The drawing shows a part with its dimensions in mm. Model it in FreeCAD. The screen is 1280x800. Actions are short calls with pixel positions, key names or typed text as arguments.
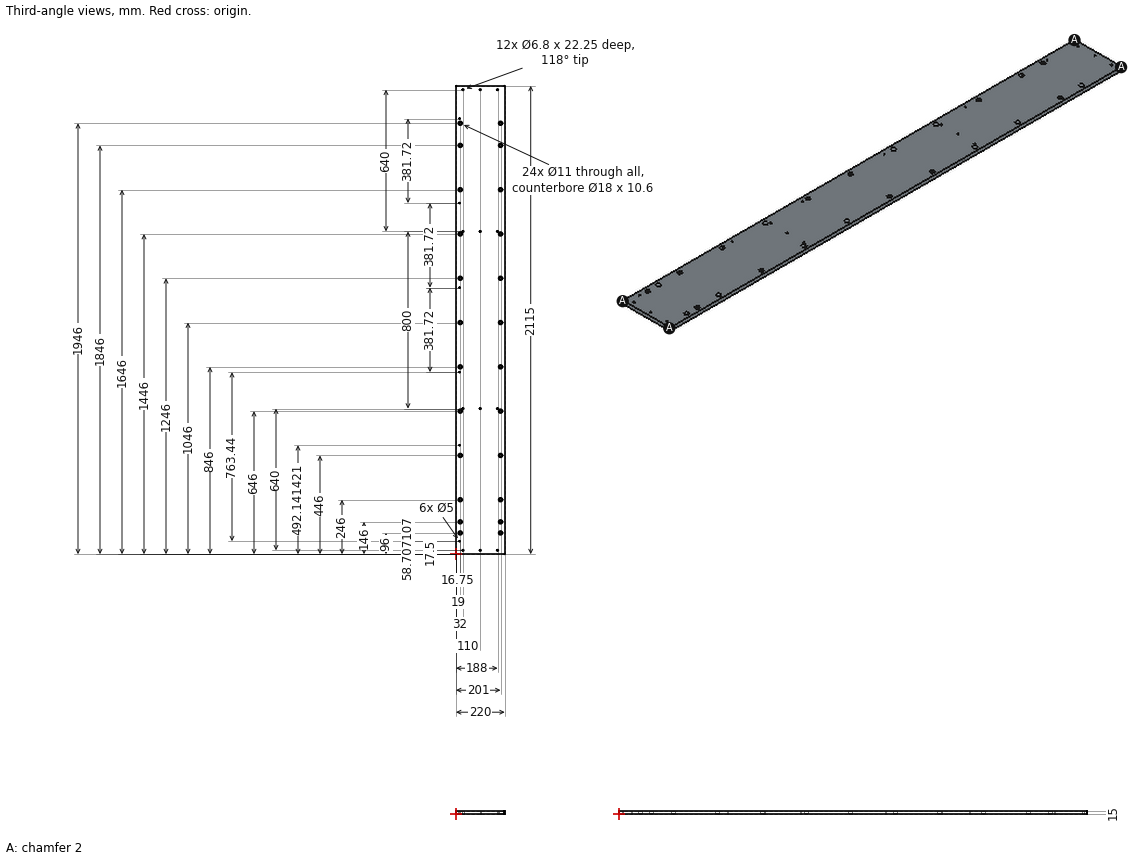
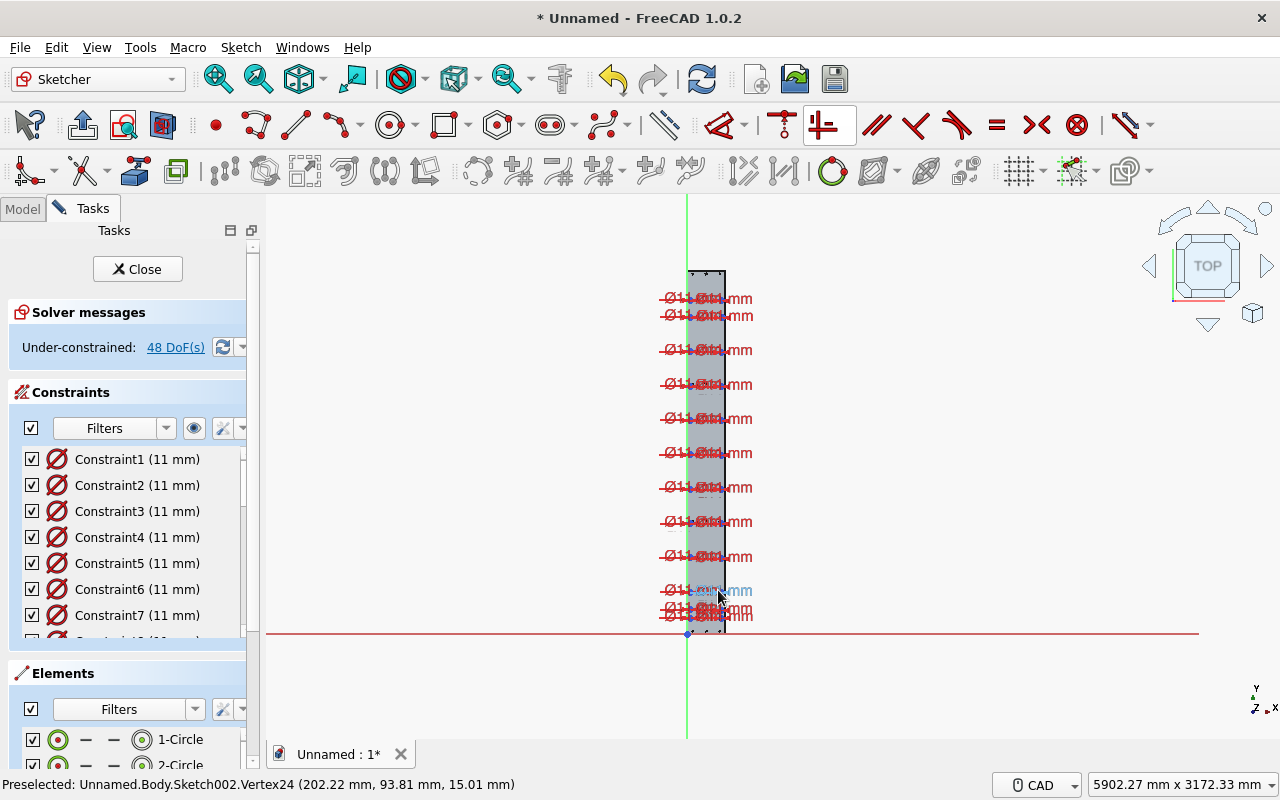
click(690, 300)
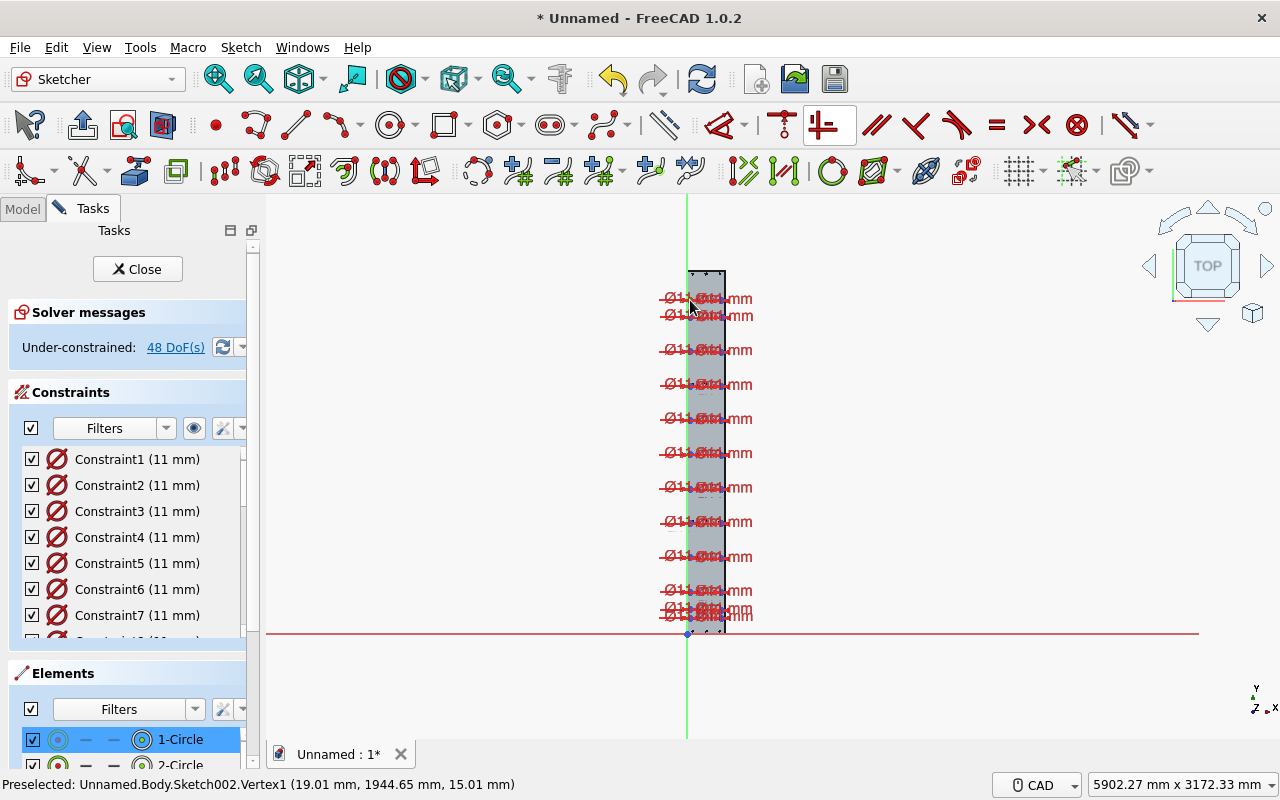
click(721, 301)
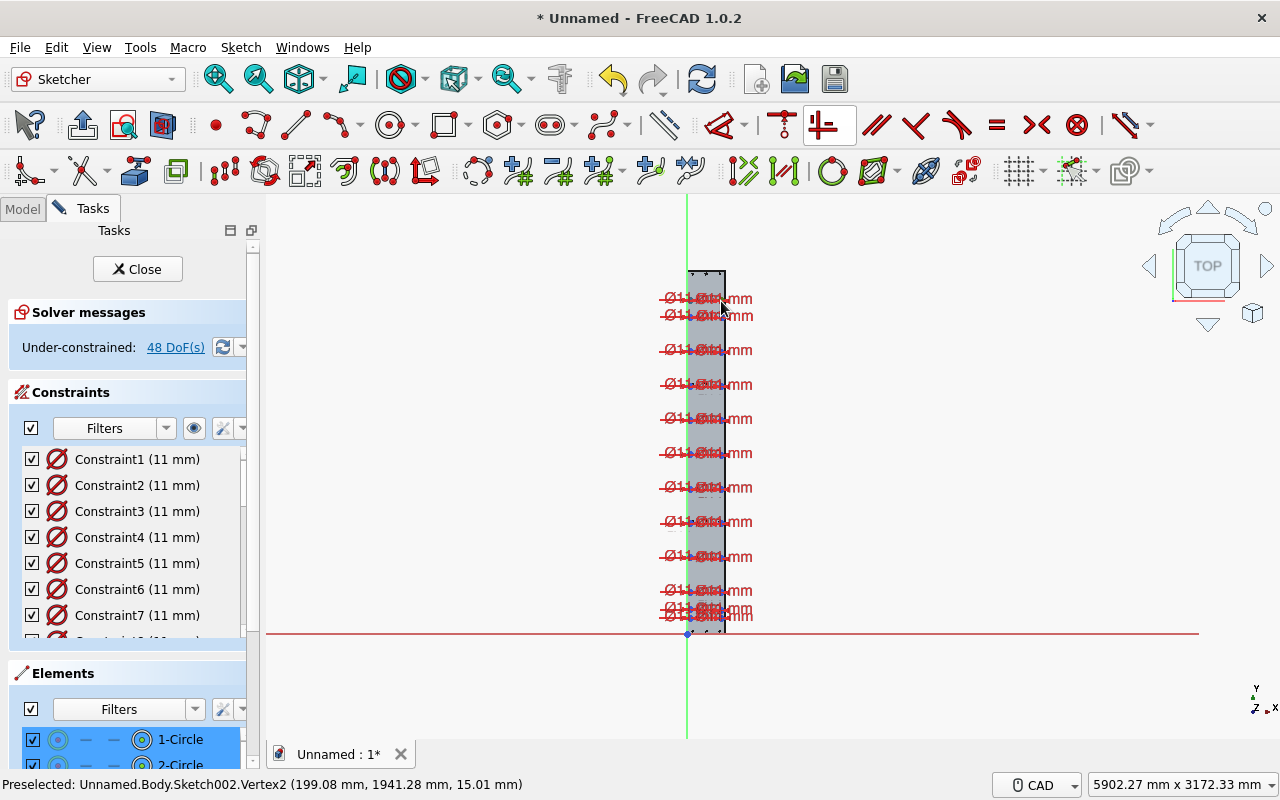
key(h)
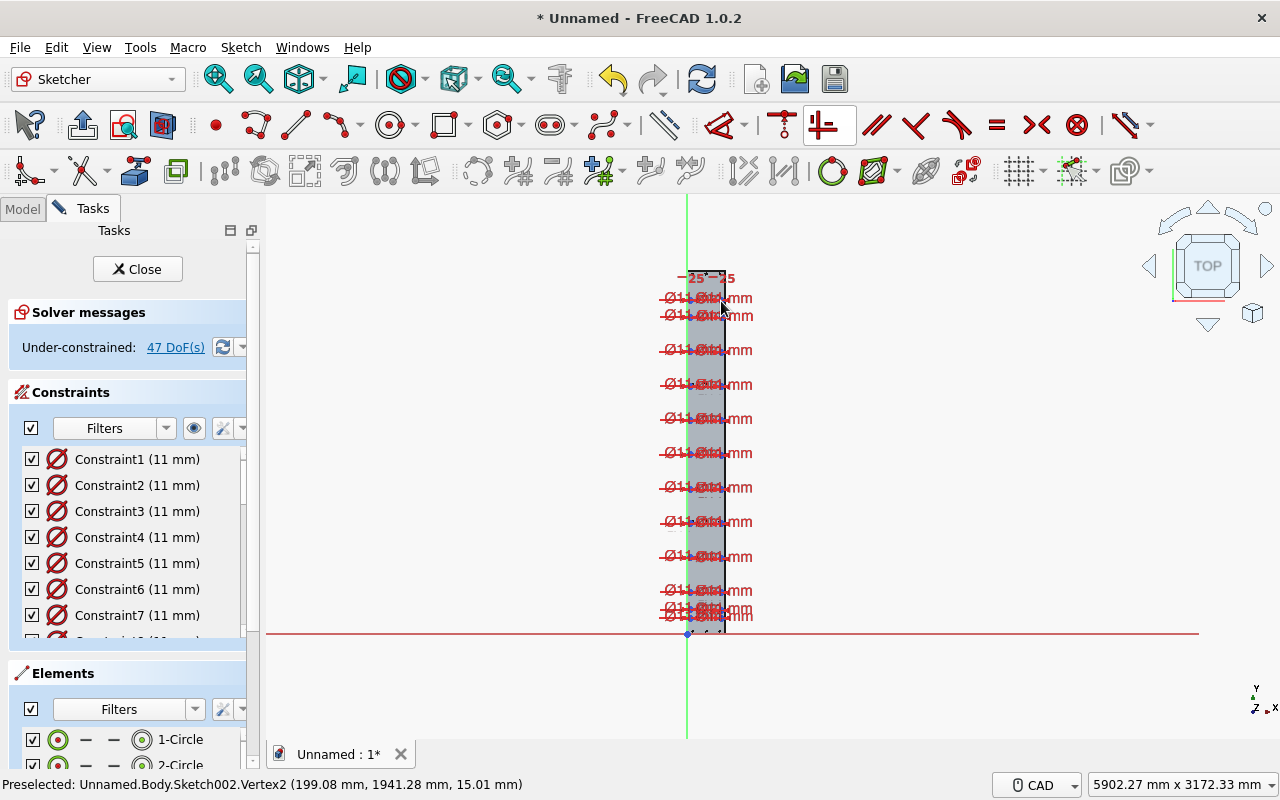
click(690, 300)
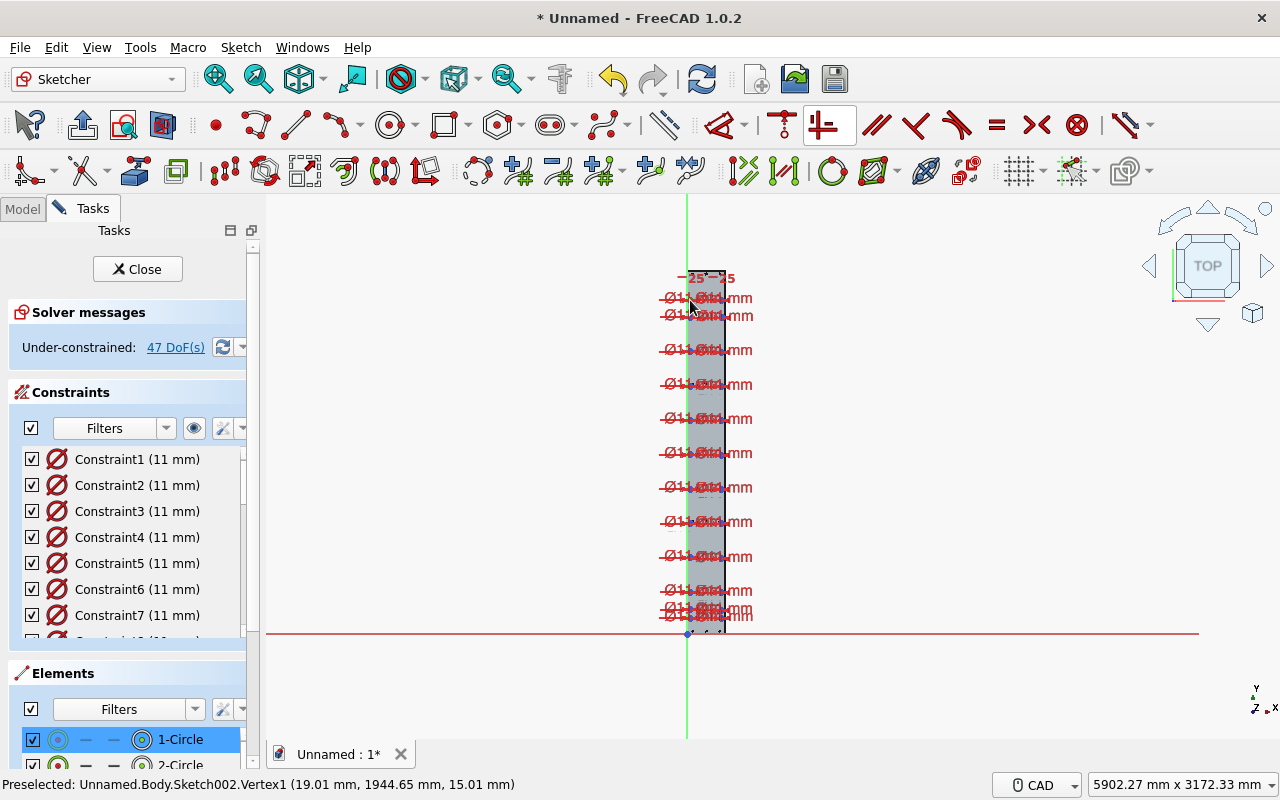
click(690, 317)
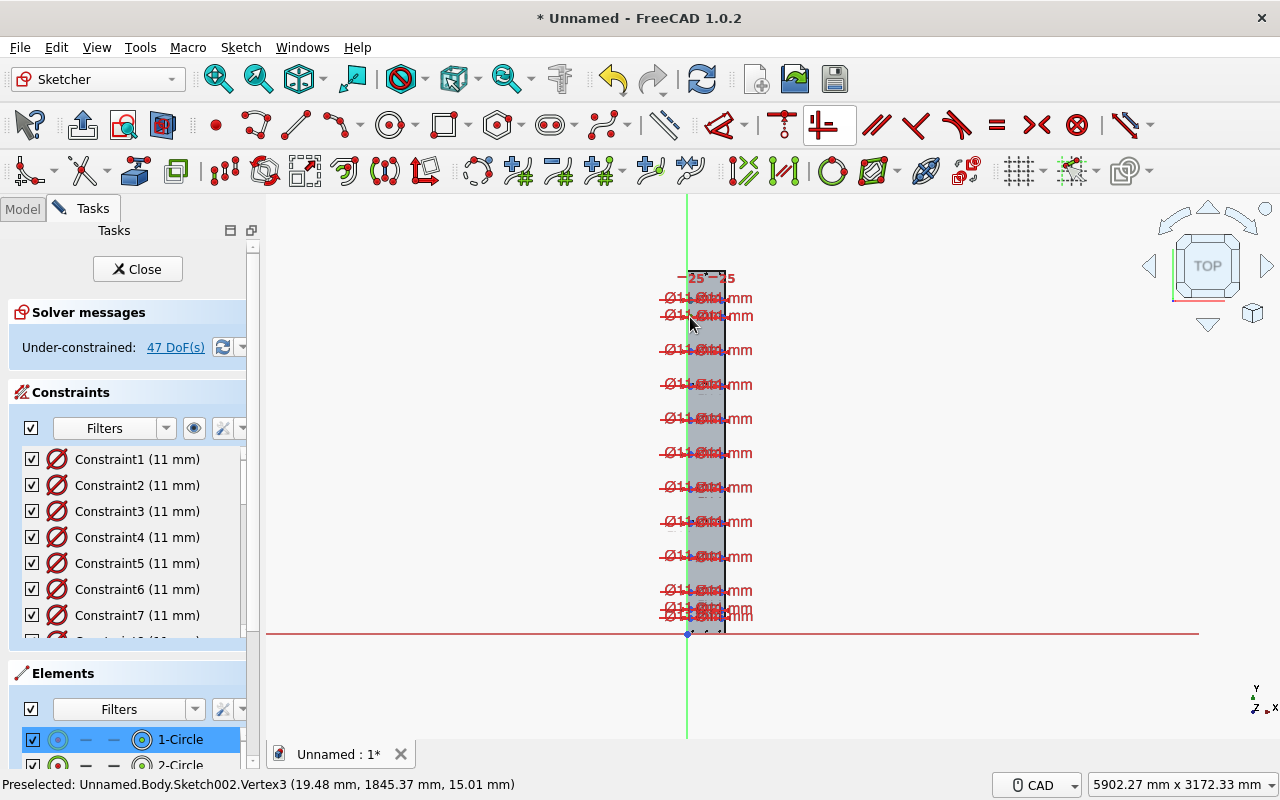
click(850, 126)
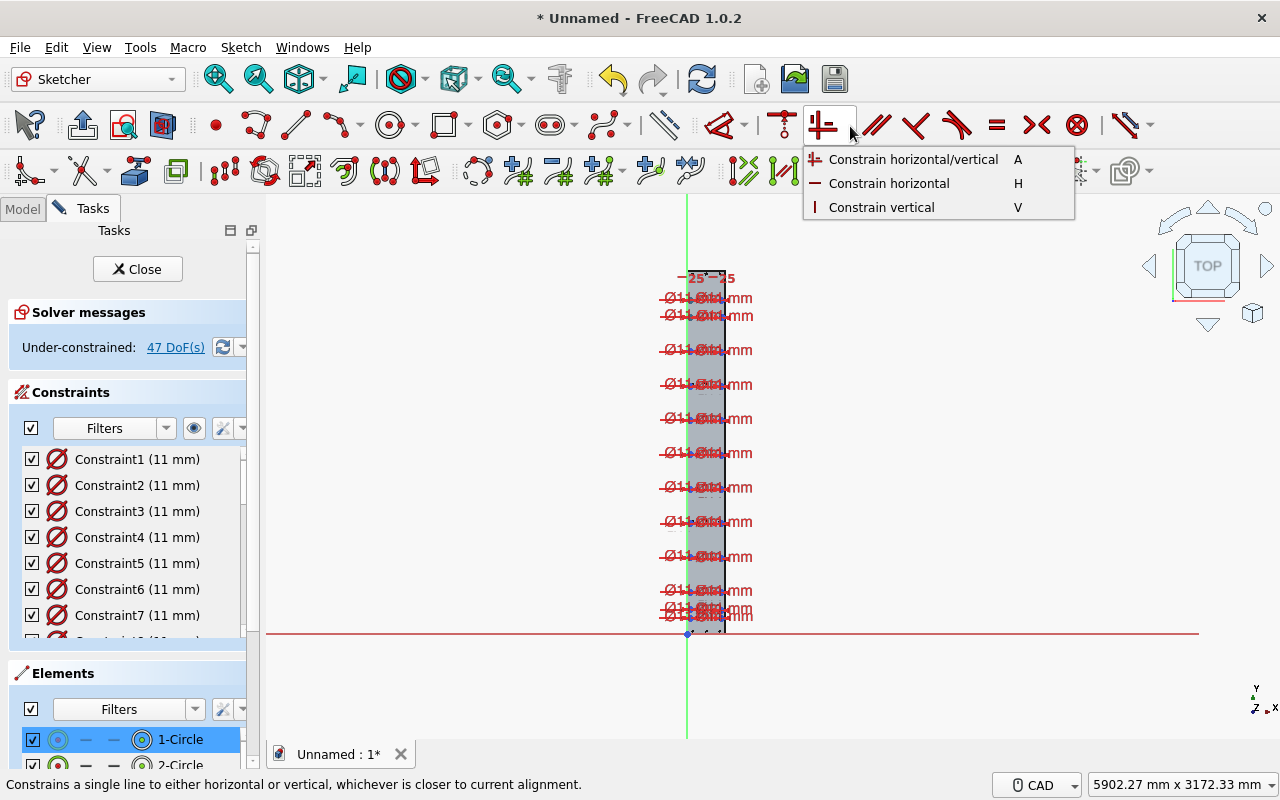
click(939, 207)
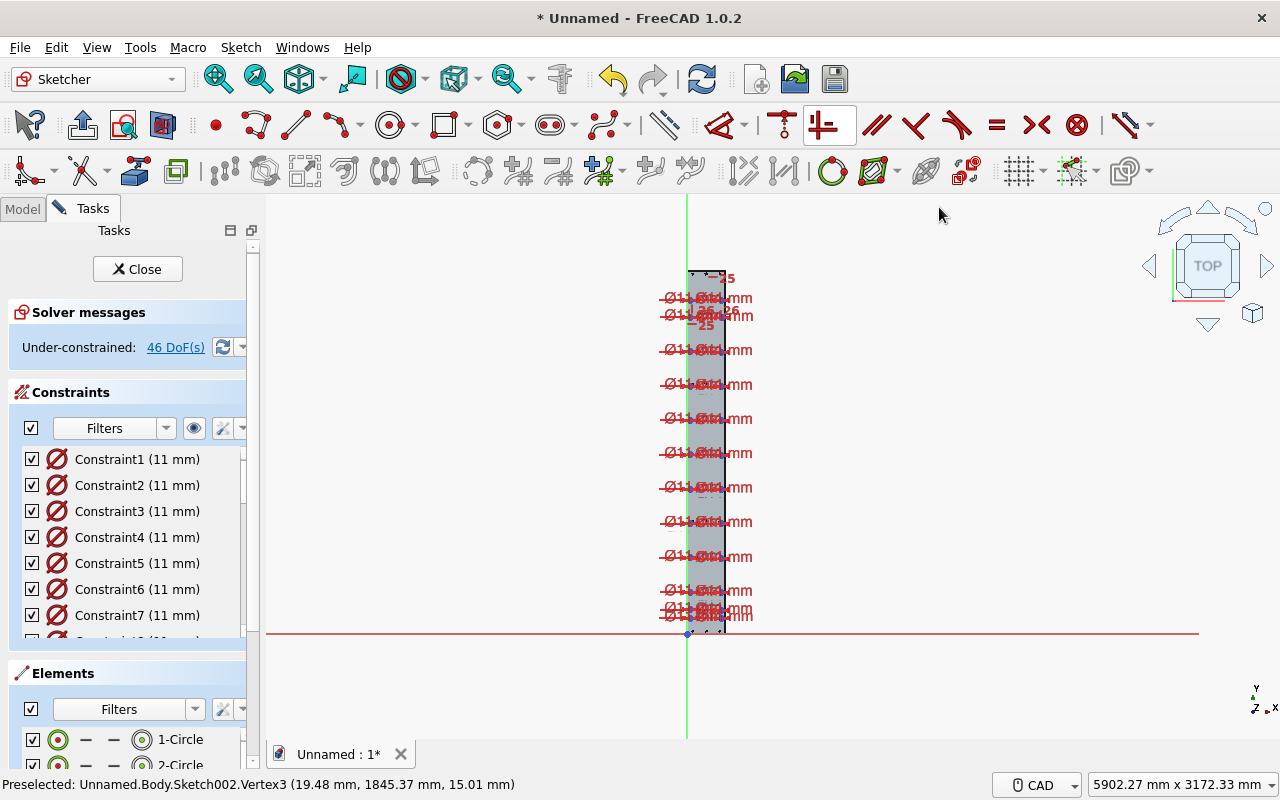
click(721, 300)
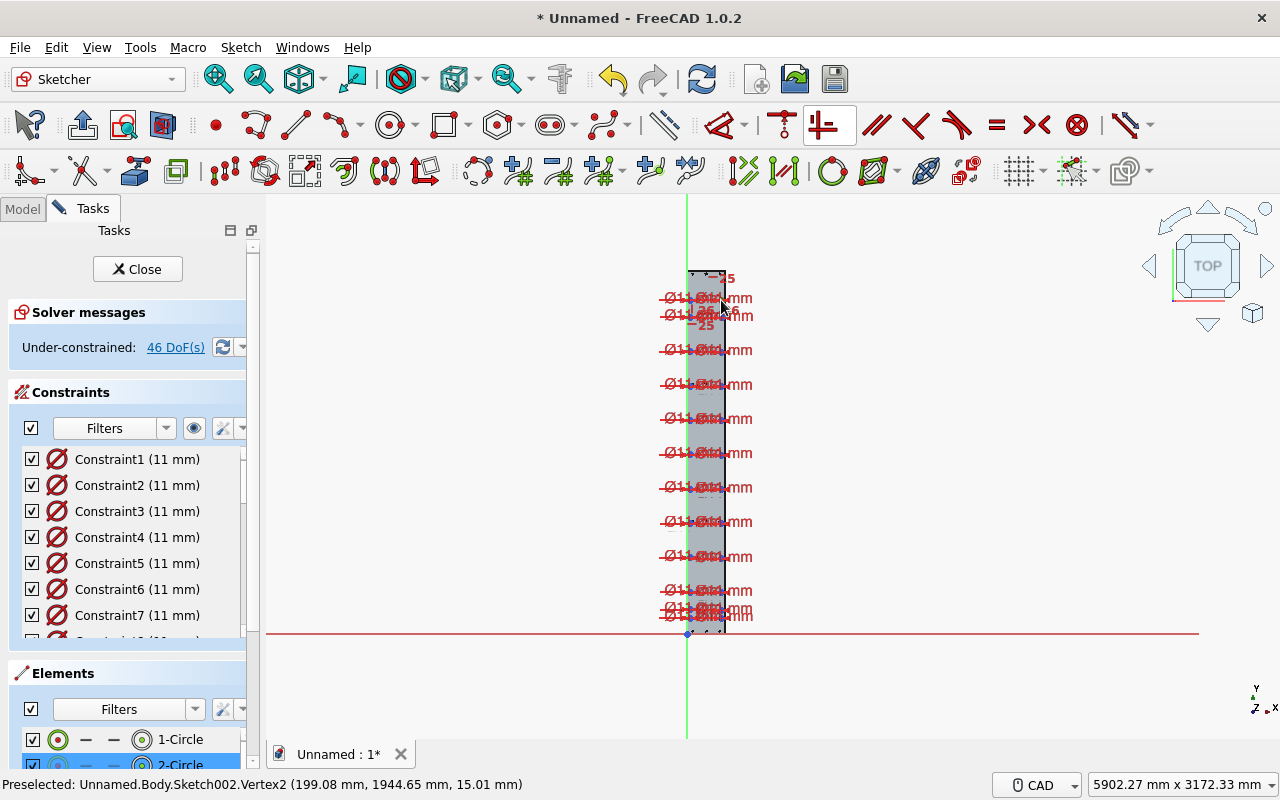
scroll(722, 318, up, 4)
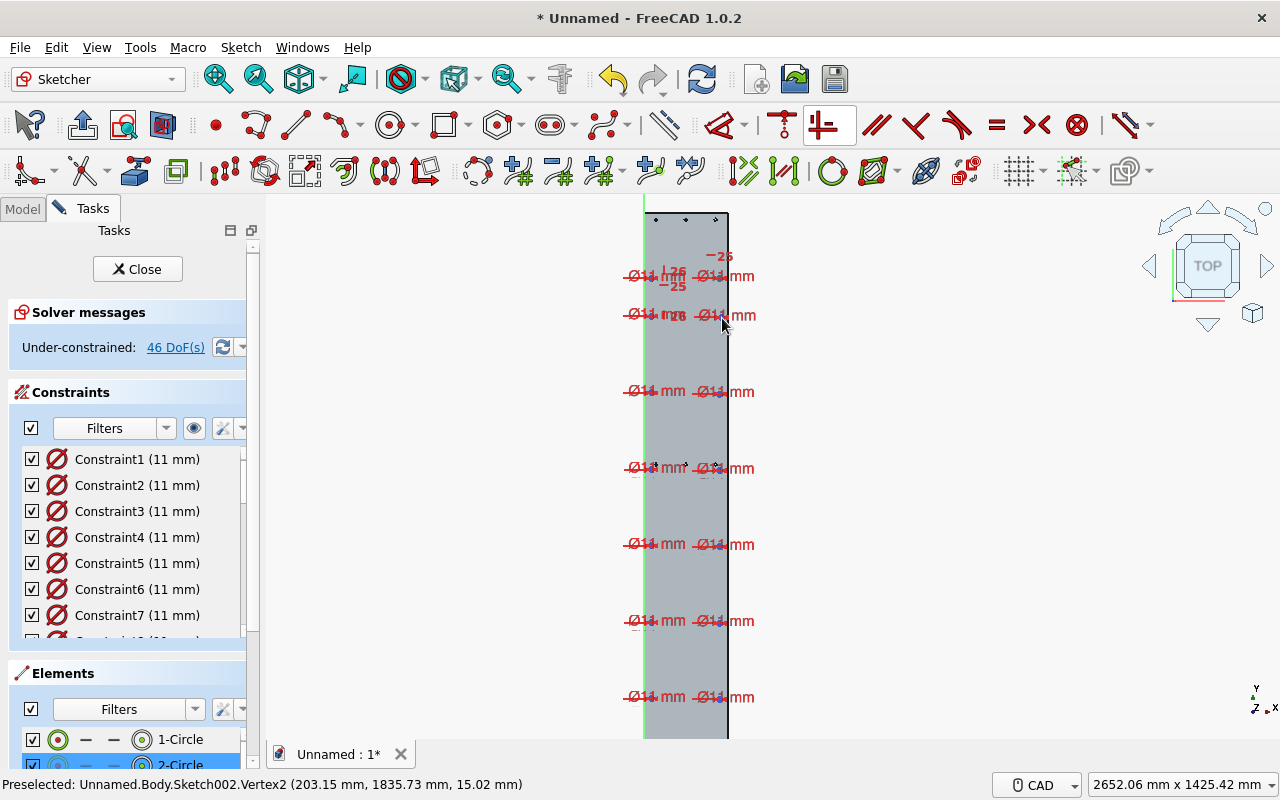
click(722, 317)